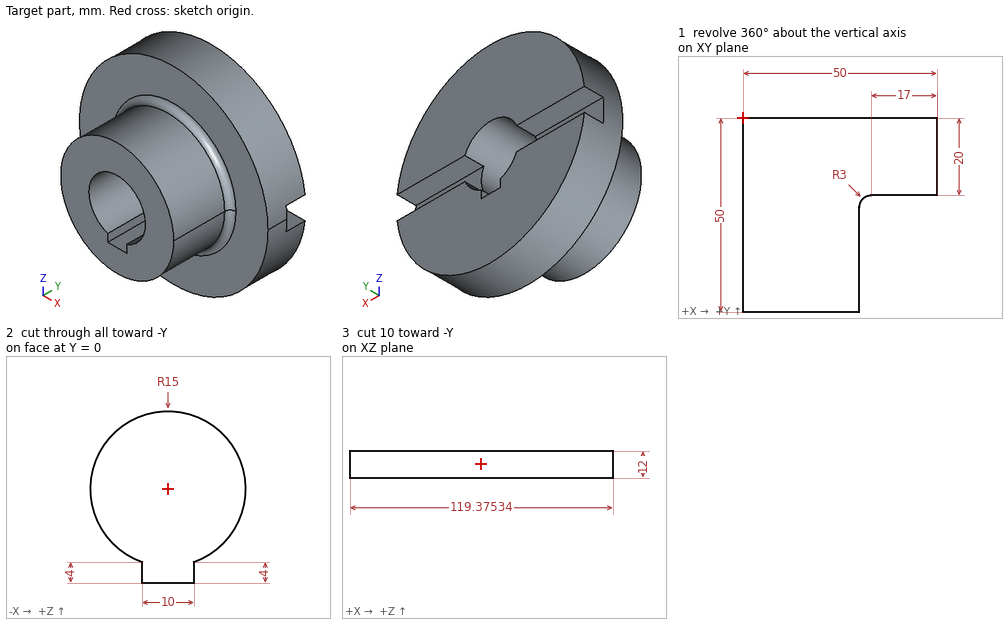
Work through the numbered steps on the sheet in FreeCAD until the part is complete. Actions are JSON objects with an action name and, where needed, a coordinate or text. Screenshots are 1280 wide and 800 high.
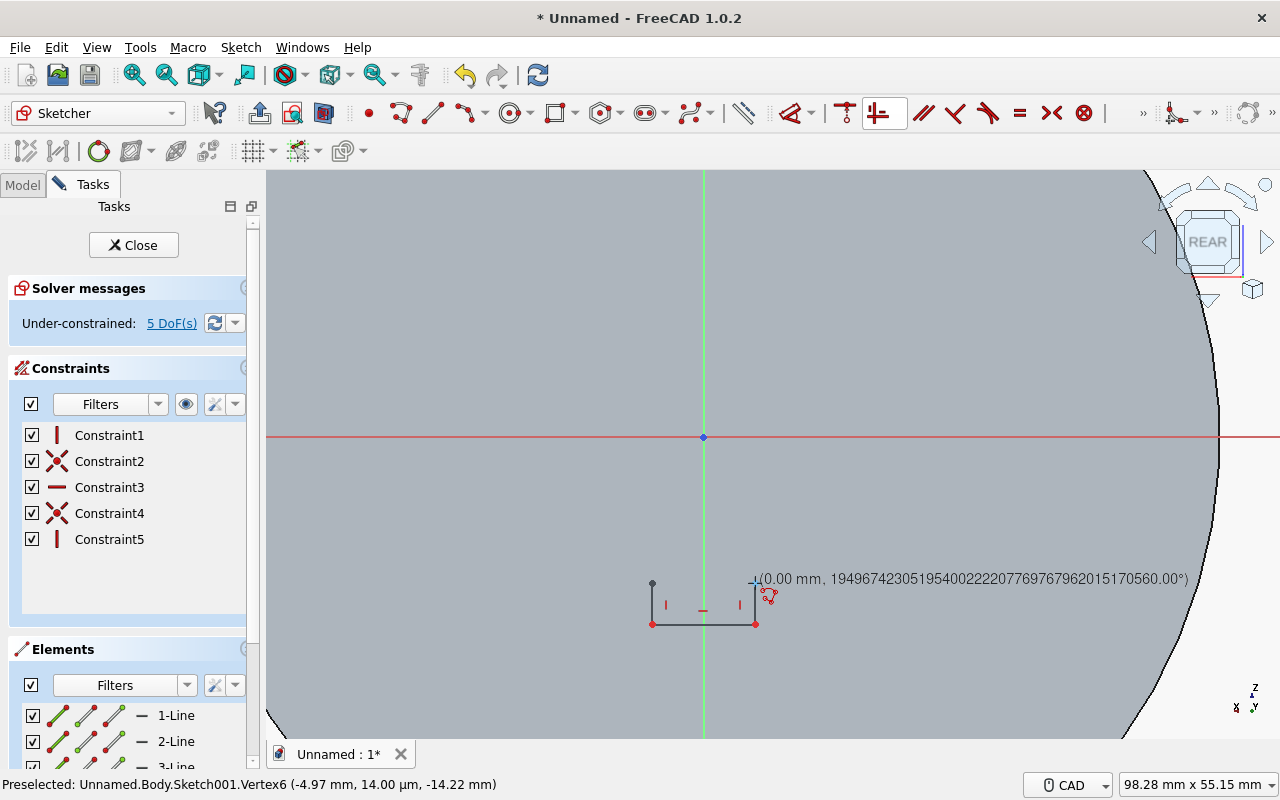
{"action": "left_click", "coordinate": [466, 114]}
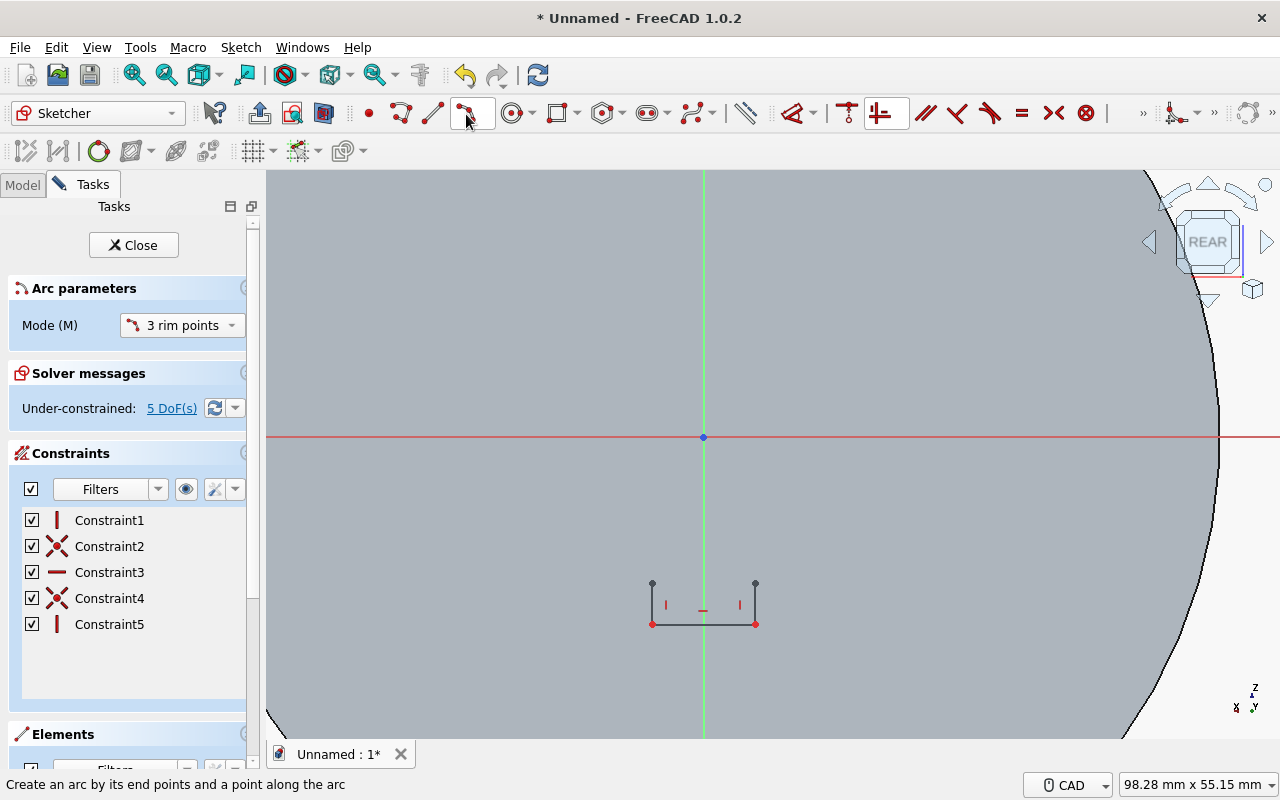
{"action": "left_click", "coordinate": [755, 584]}
{"action": "left_click", "coordinate": [652, 584]}
{"action": "left_click", "coordinate": [786, 306]}
{"action": "key", "text": "Escape"}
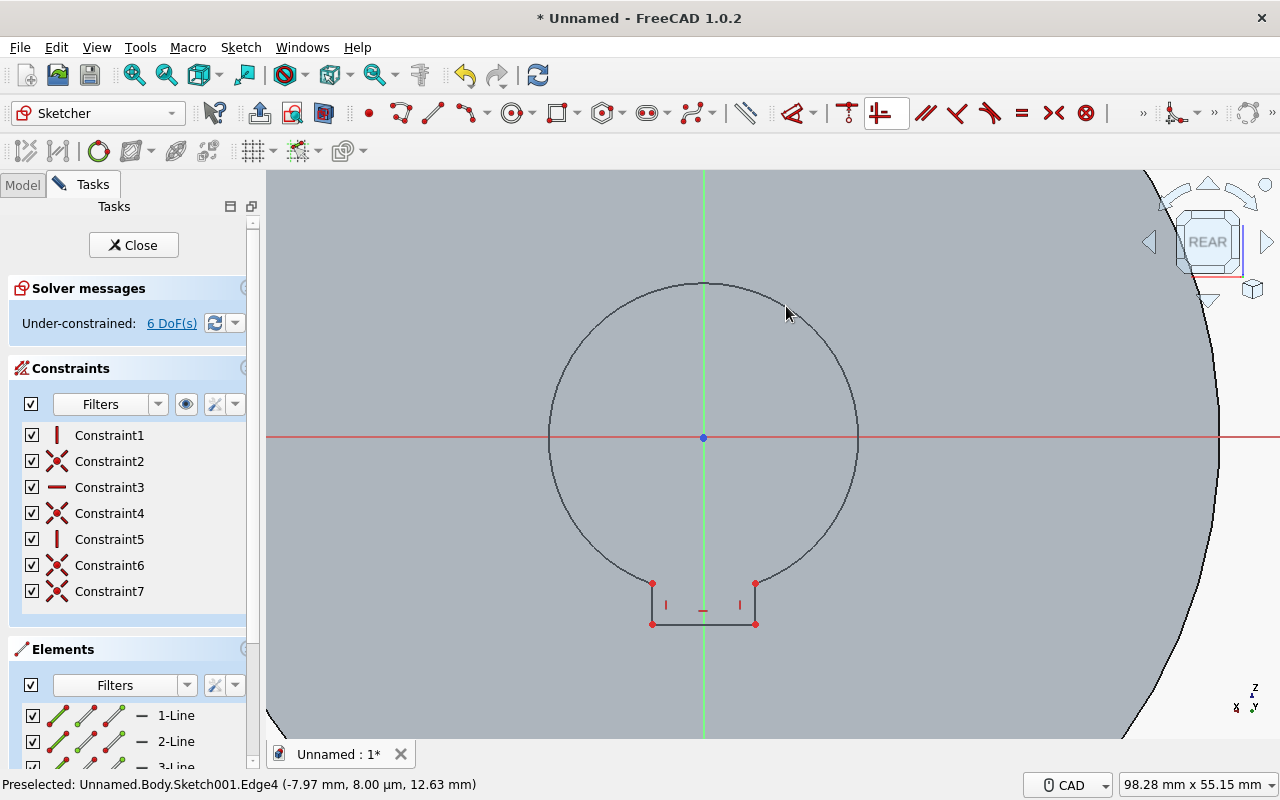
{"action": "left_click_drag", "start_coordinate": [693, 427], "coordinate": [714, 448]}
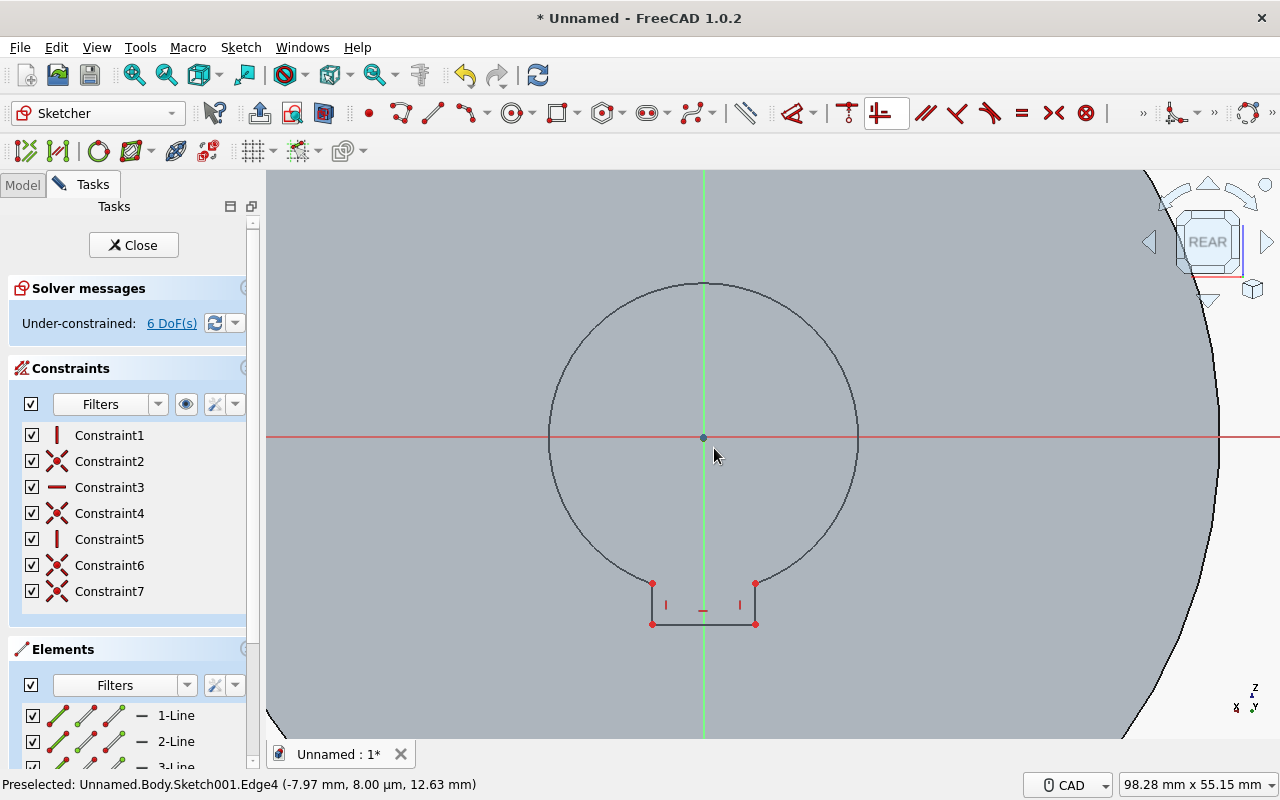
{"action": "left_click", "coordinate": [848, 114]}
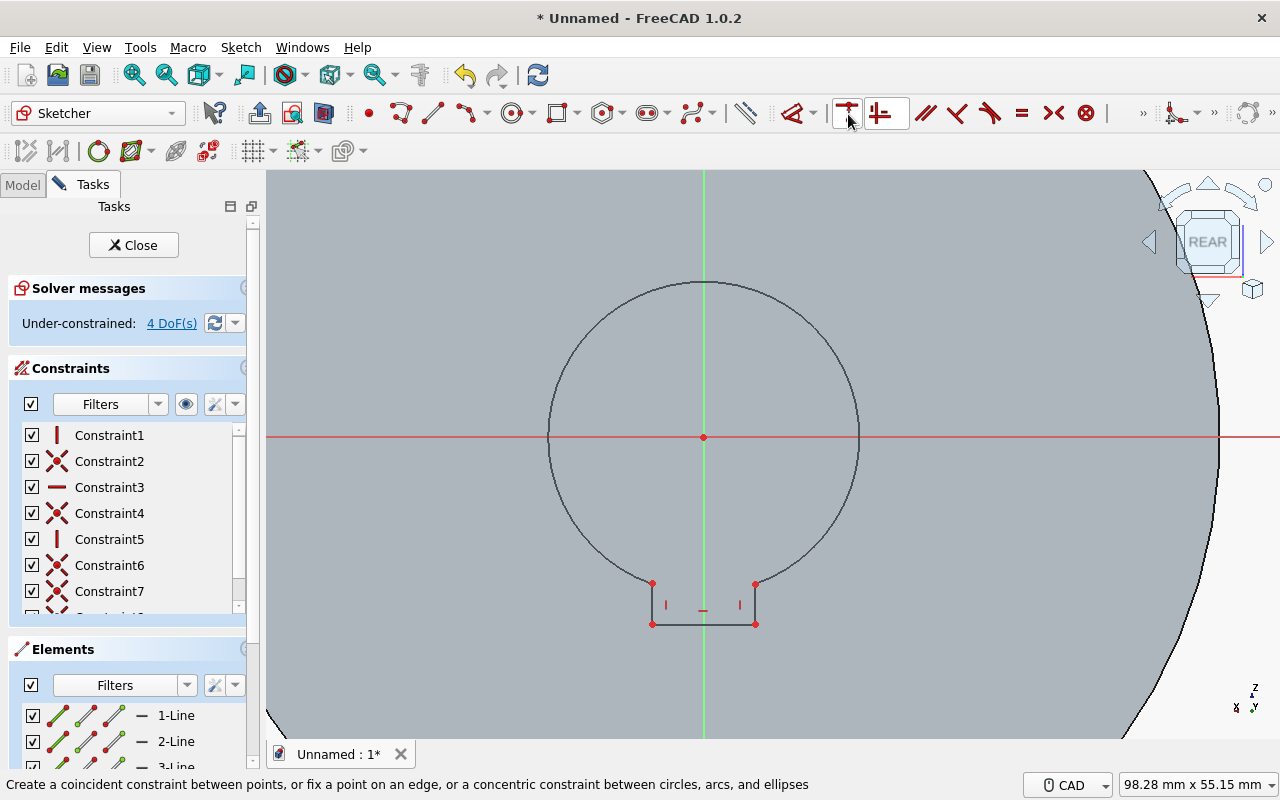
{"action": "left_click", "coordinate": [792, 114]}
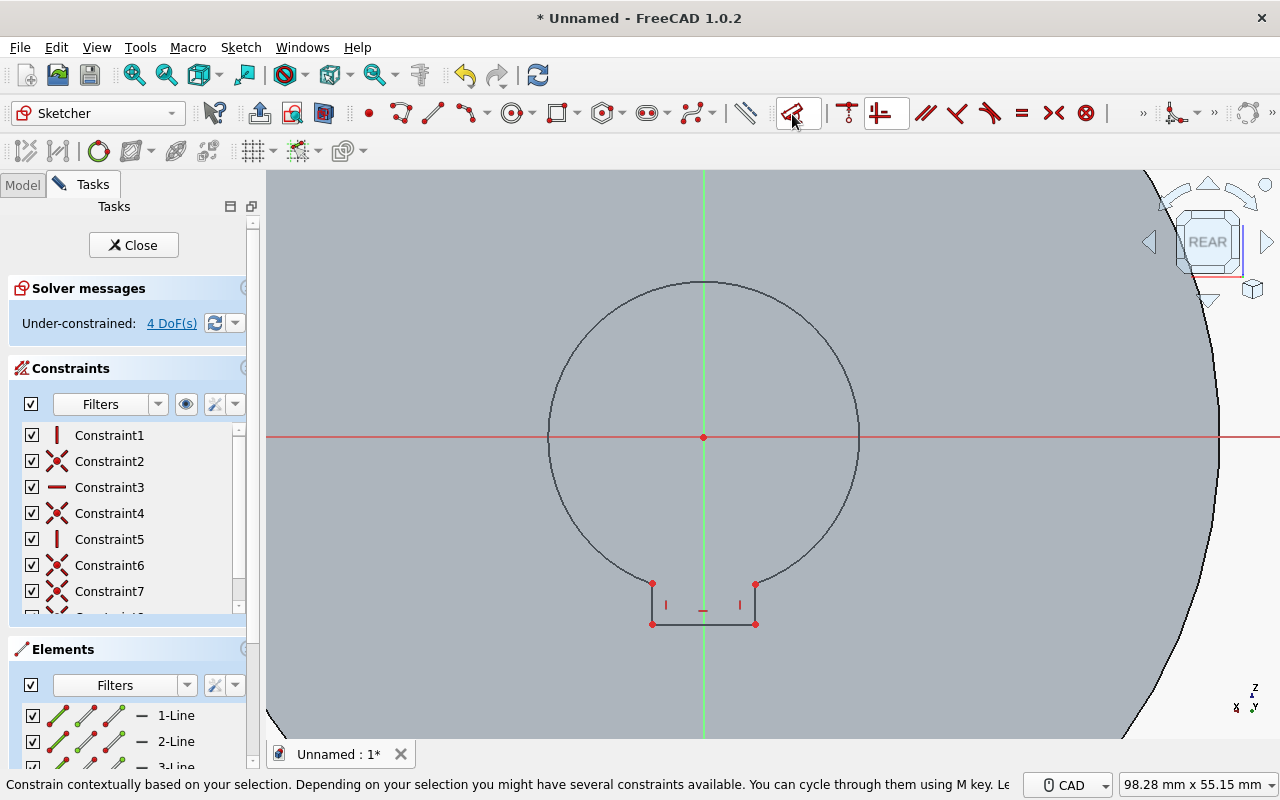
{"action": "left_click", "coordinate": [844, 370]}
{"action": "left_click", "coordinate": [873, 356]}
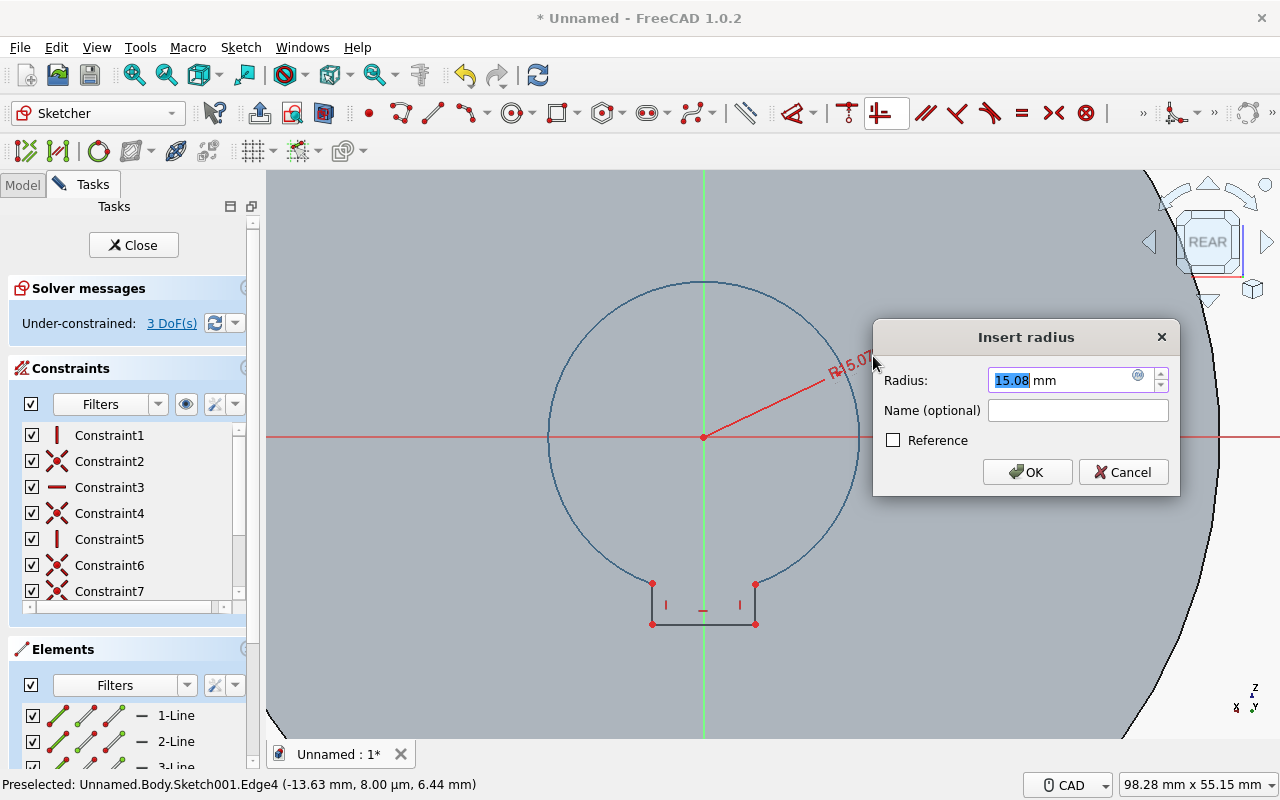
{"action": "type", "text": "15"}
{"action": "key", "text": "Return"}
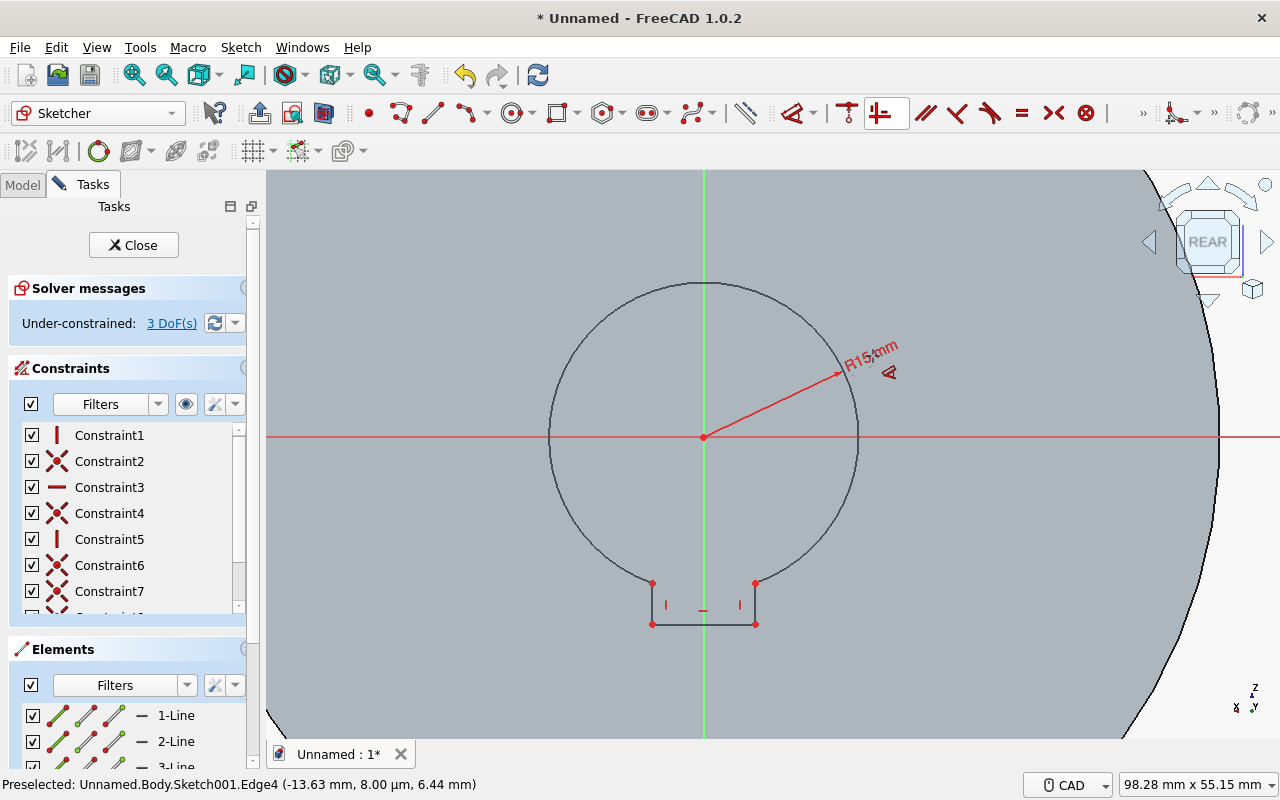
{"action": "left_click", "coordinate": [652, 596]}
{"action": "left_click", "coordinate": [618, 604]}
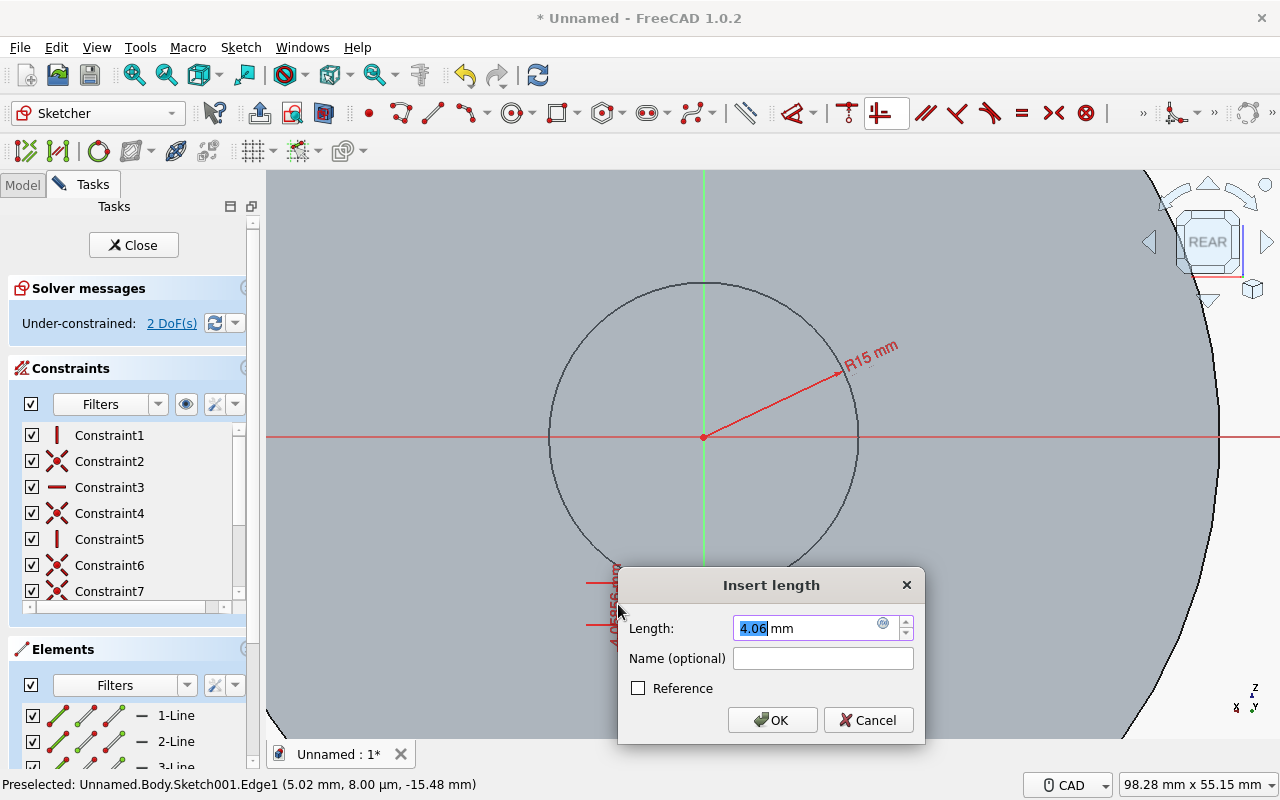
{"action": "type", "text": "4"}
{"action": "key", "text": "Return"}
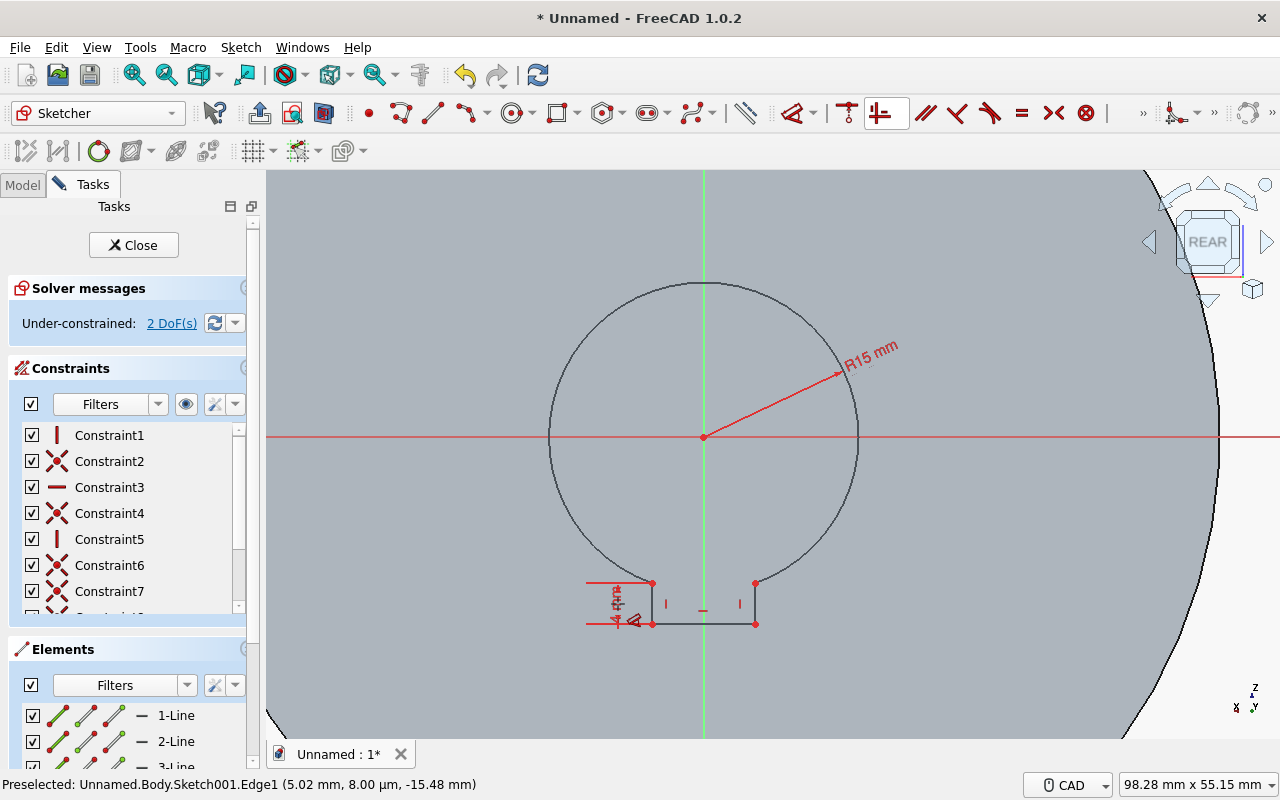
{"action": "left_click", "coordinate": [755, 612]}
{"action": "left_click", "coordinate": [789, 604]}